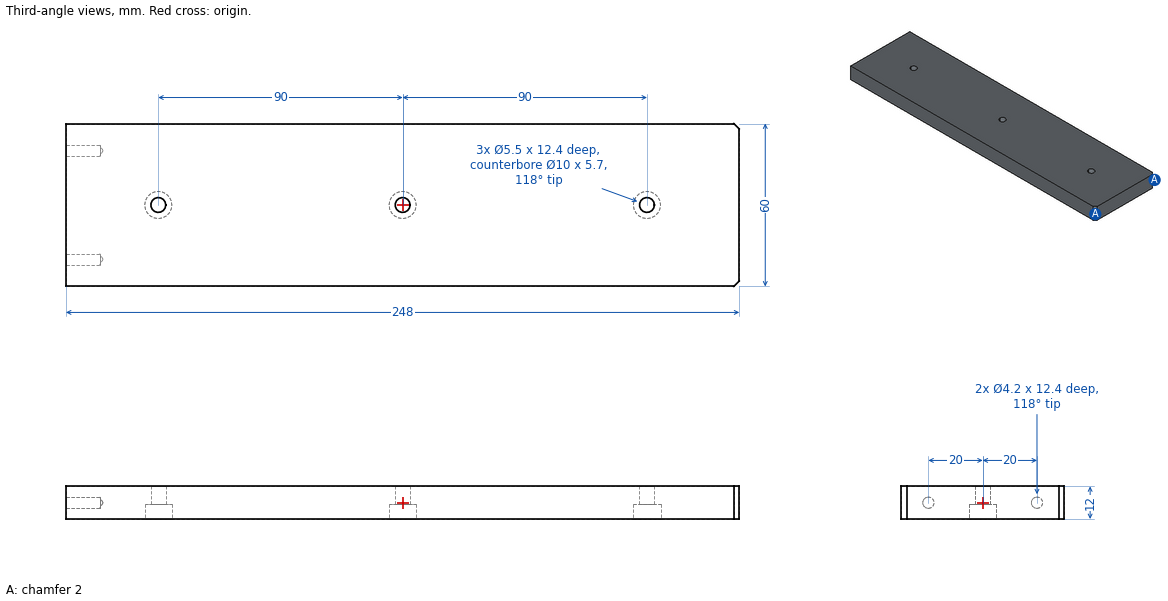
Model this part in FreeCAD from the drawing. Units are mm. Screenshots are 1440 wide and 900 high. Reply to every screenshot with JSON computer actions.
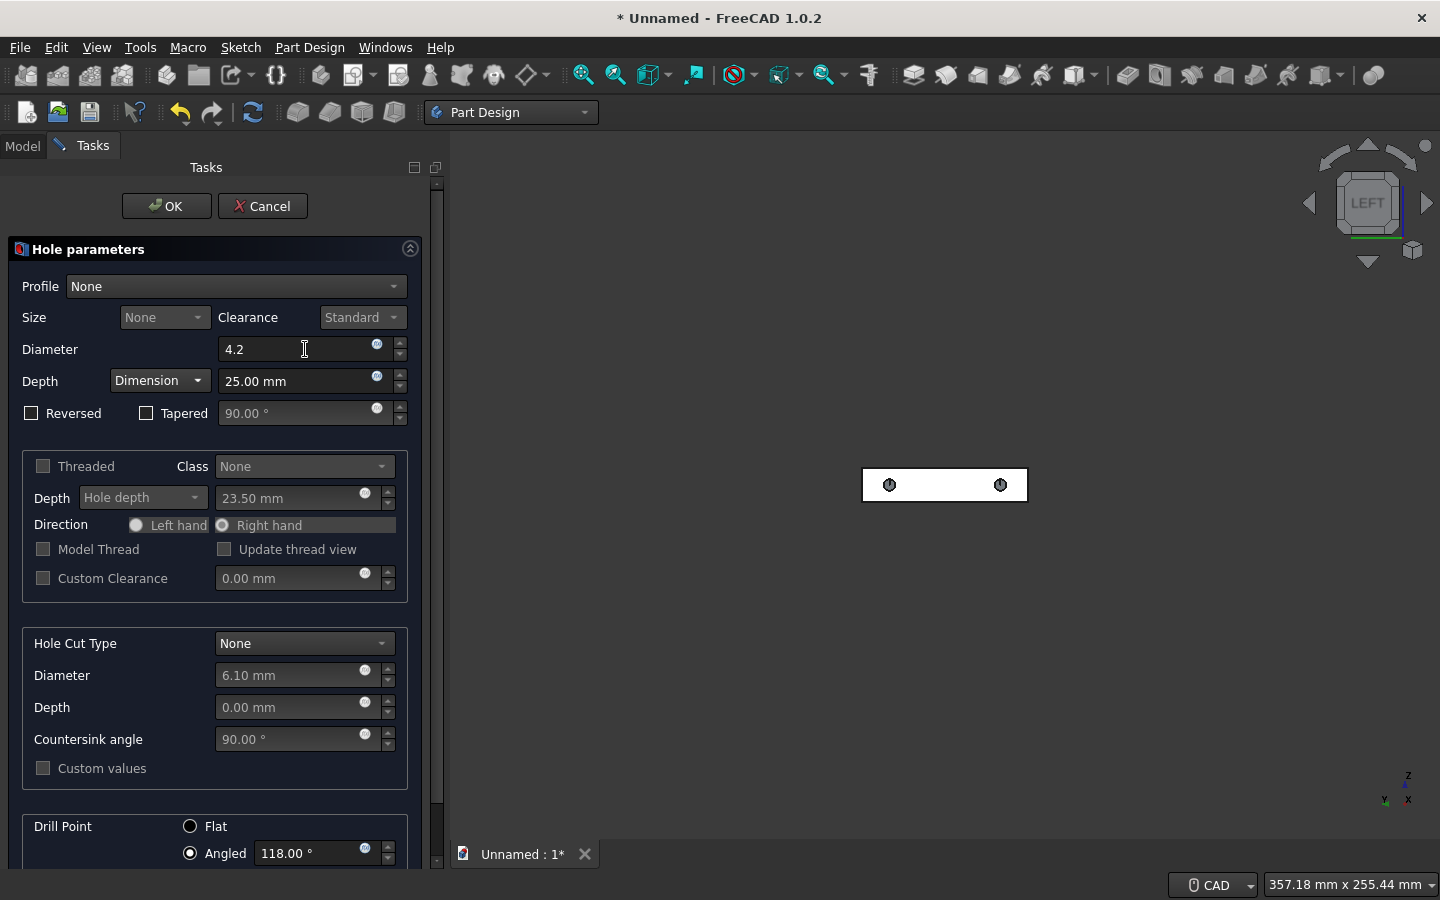
{"action": "triple_click", "coordinate": [305, 381]}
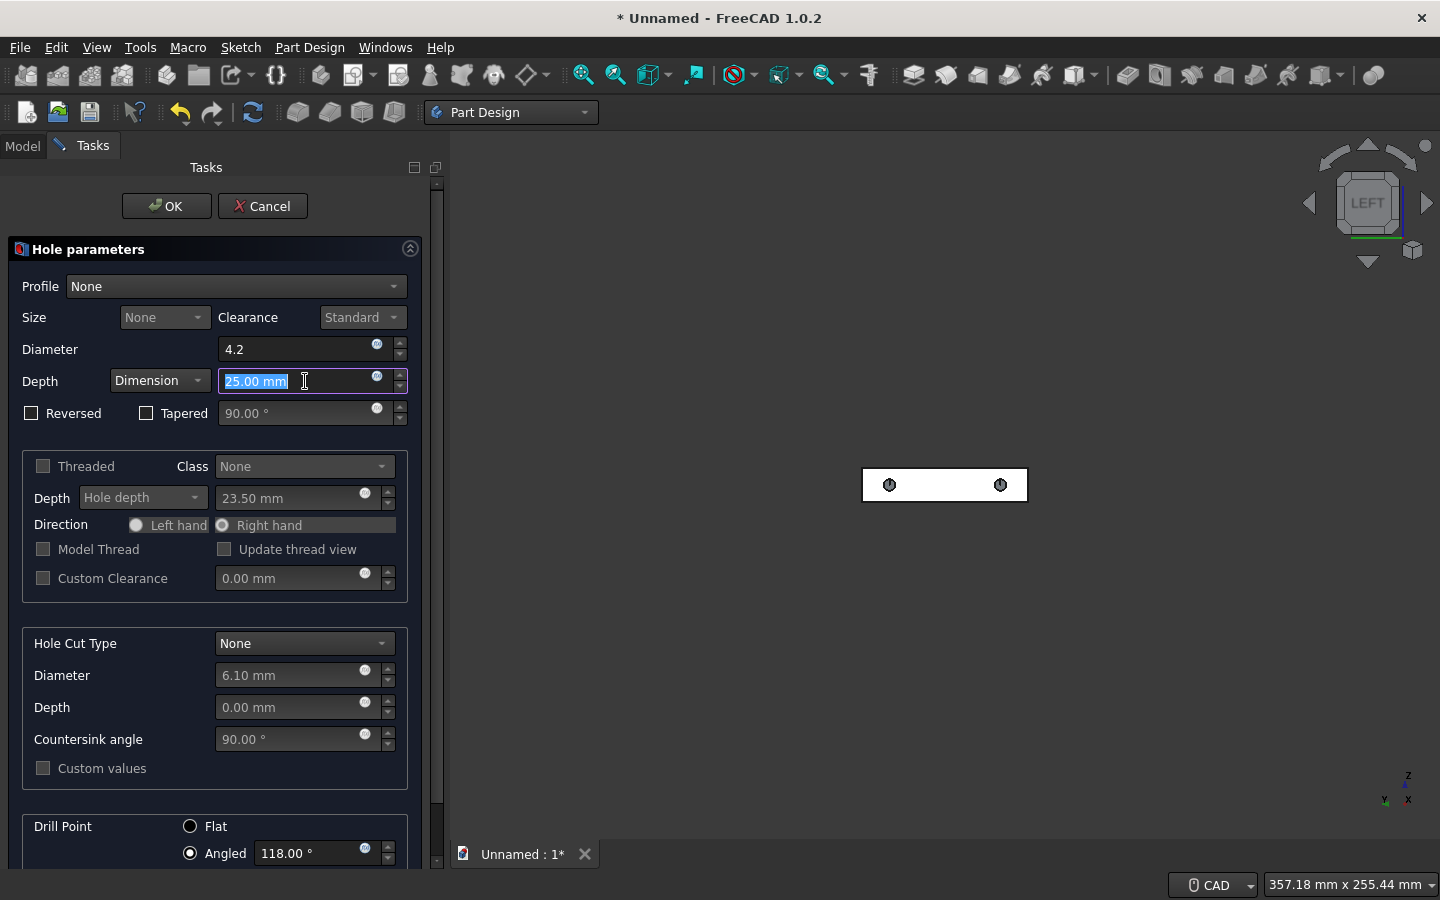
{"action": "type", "text": "12.4"}
{"action": "key", "text": "Tab"}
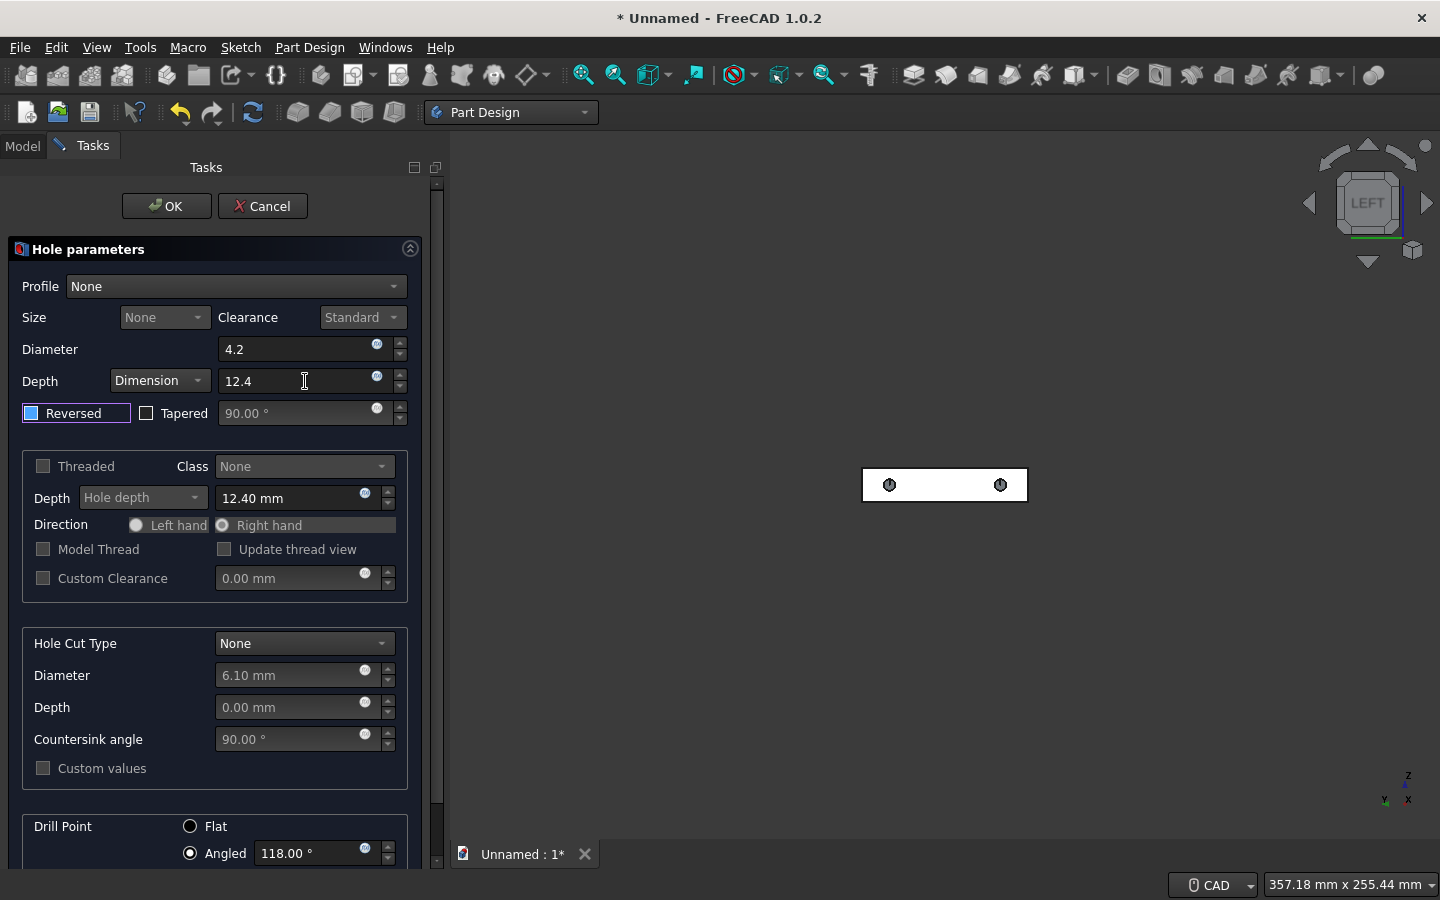
{"action": "left_click", "coordinate": [167, 206]}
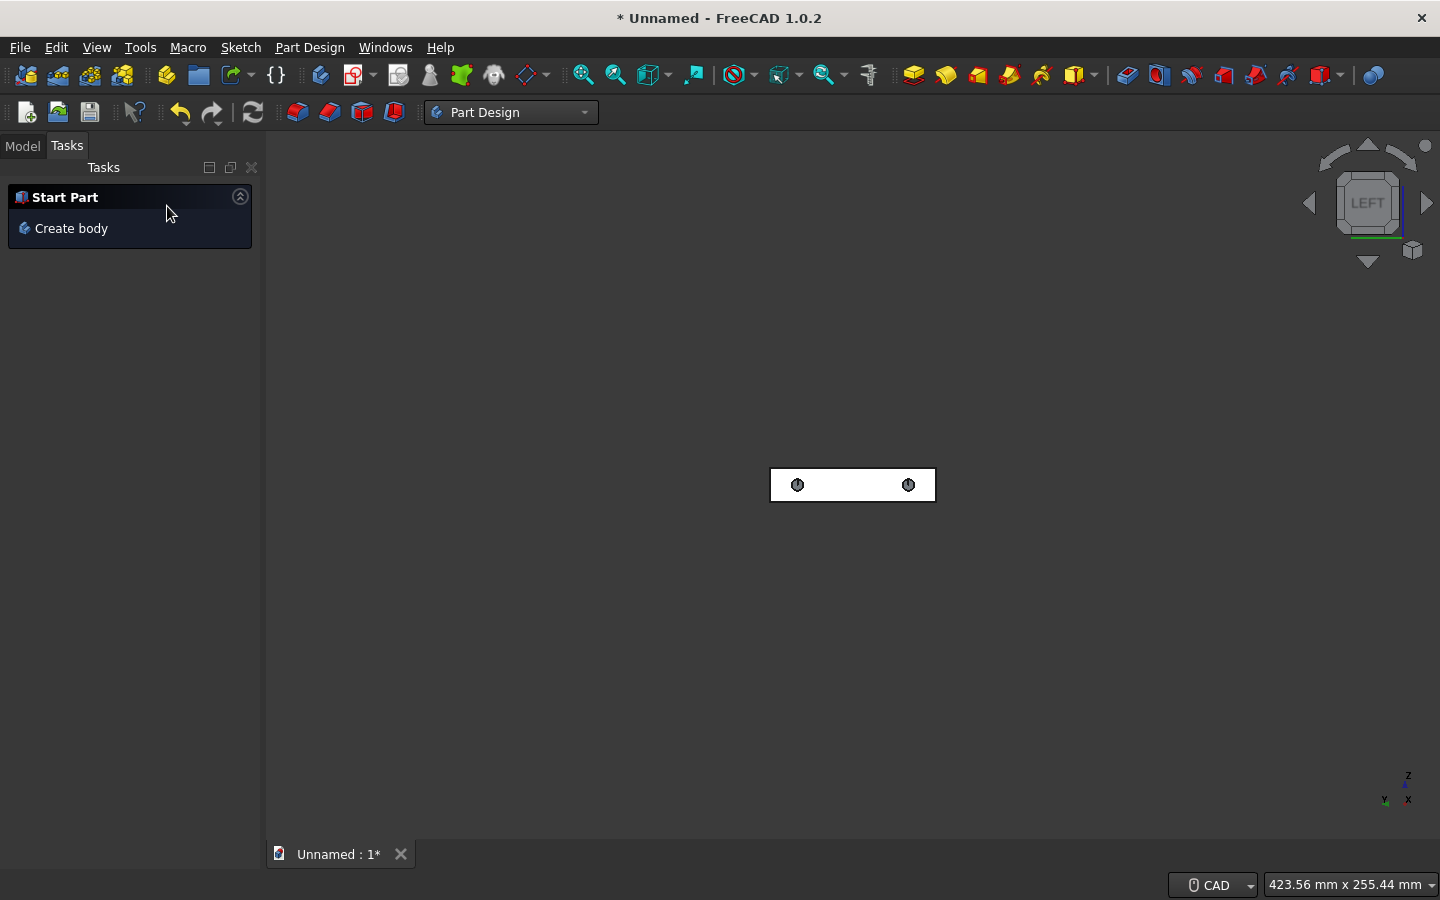
{"action": "left_click", "coordinate": [584, 76]}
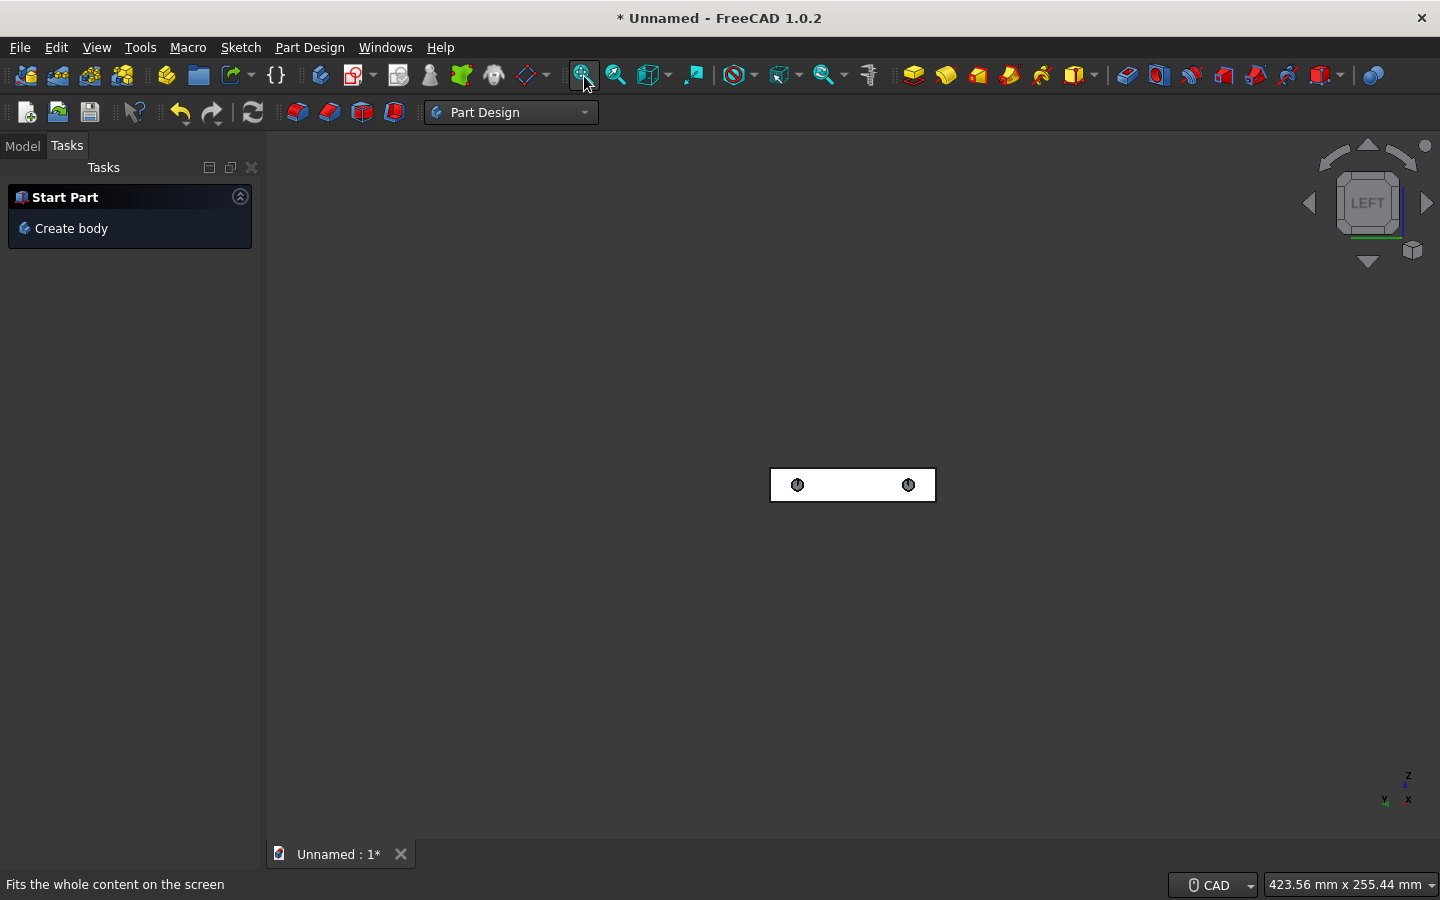
{"action": "key", "text": "0"}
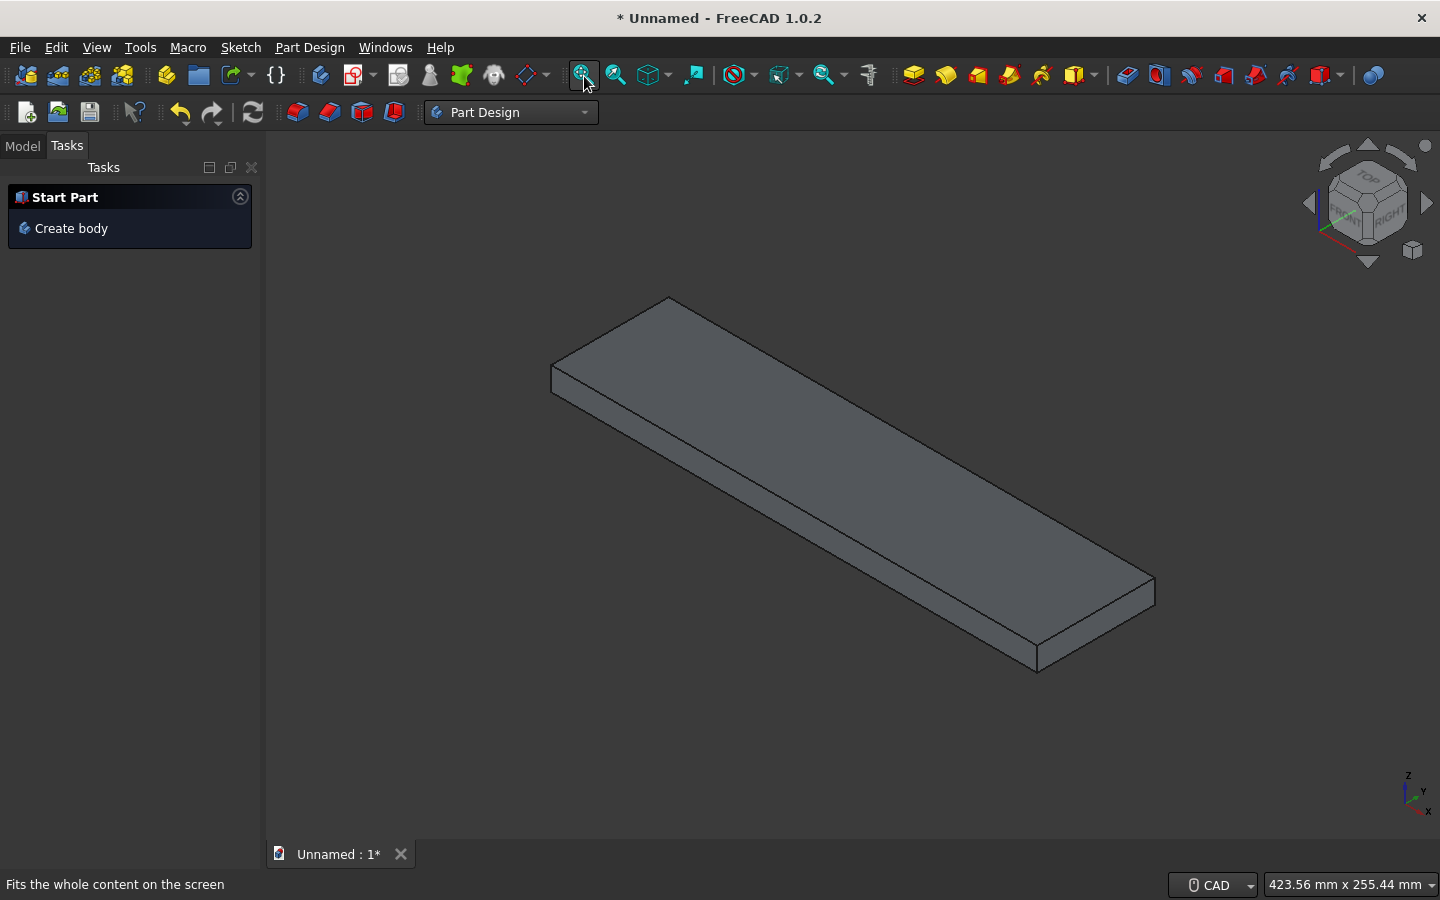
{"action": "left_click", "coordinate": [1037, 658]}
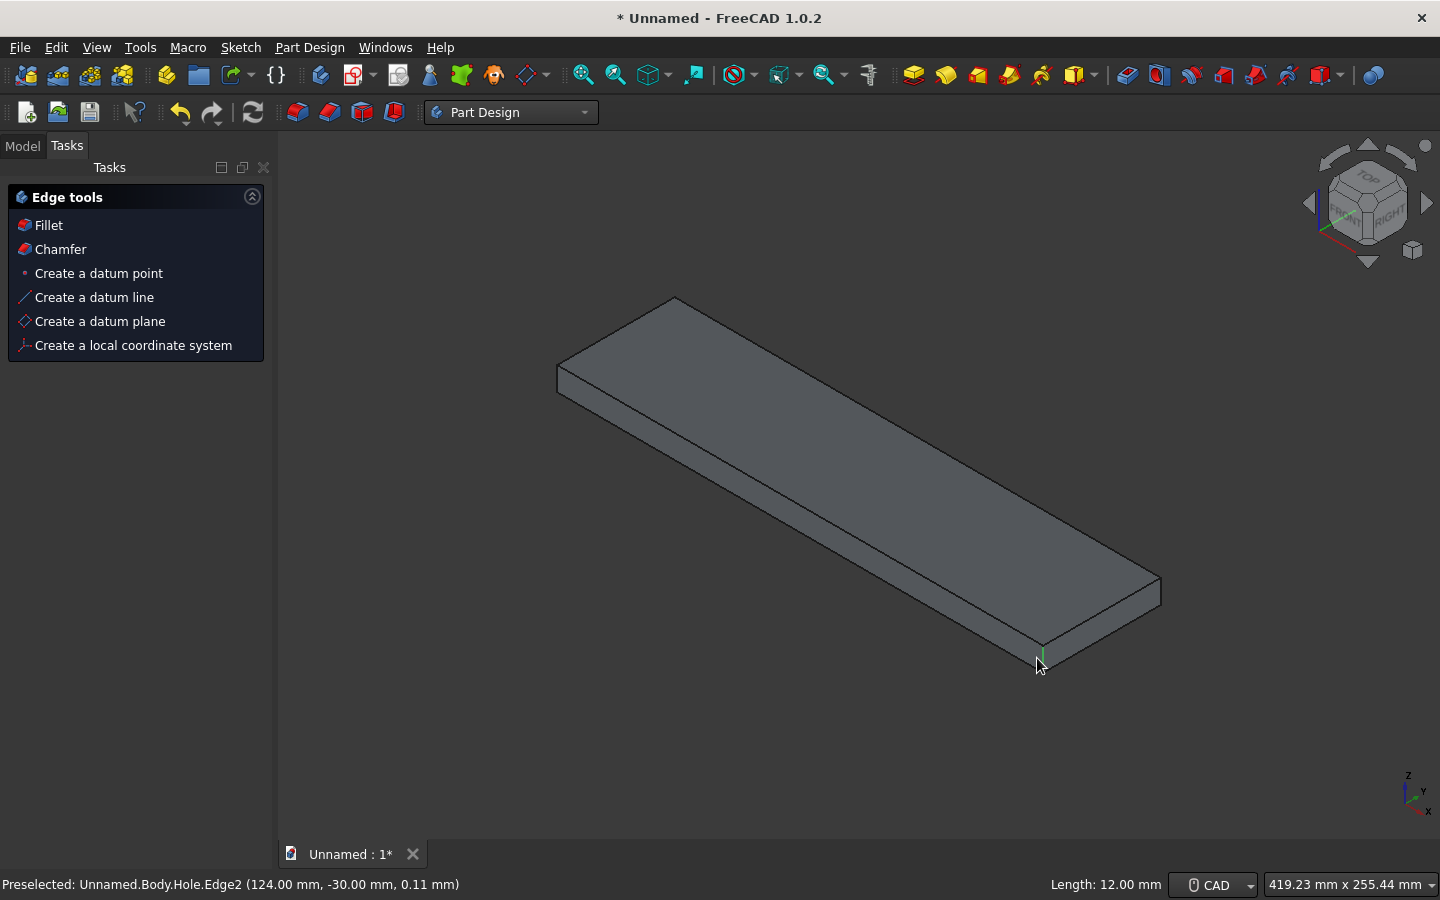
{"action": "key", "text": "2"}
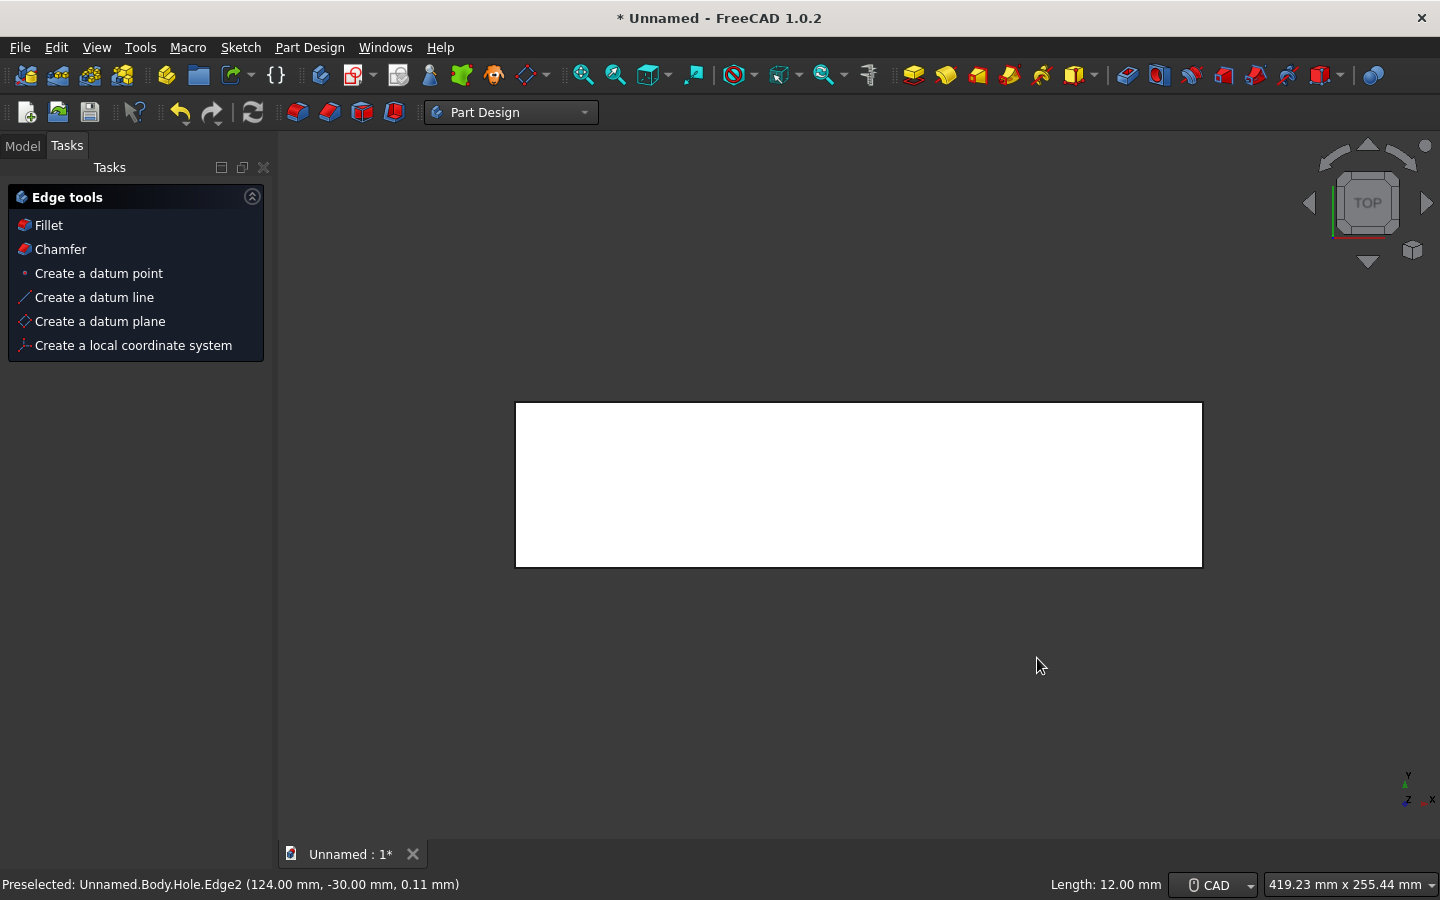
{"action": "key", "text": "1"}